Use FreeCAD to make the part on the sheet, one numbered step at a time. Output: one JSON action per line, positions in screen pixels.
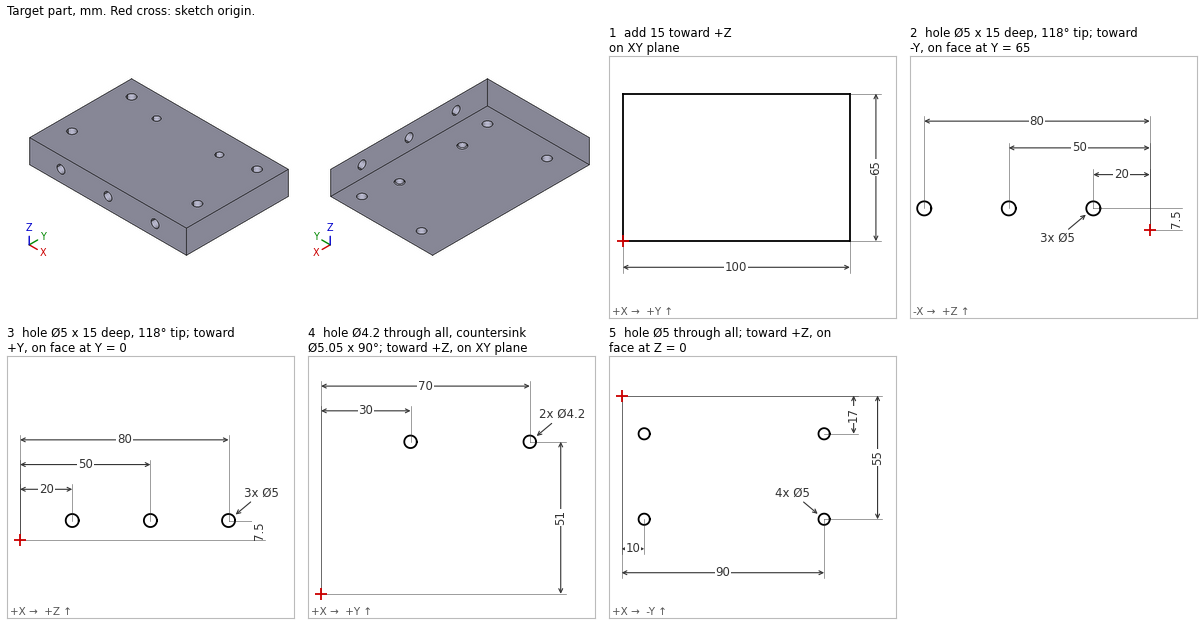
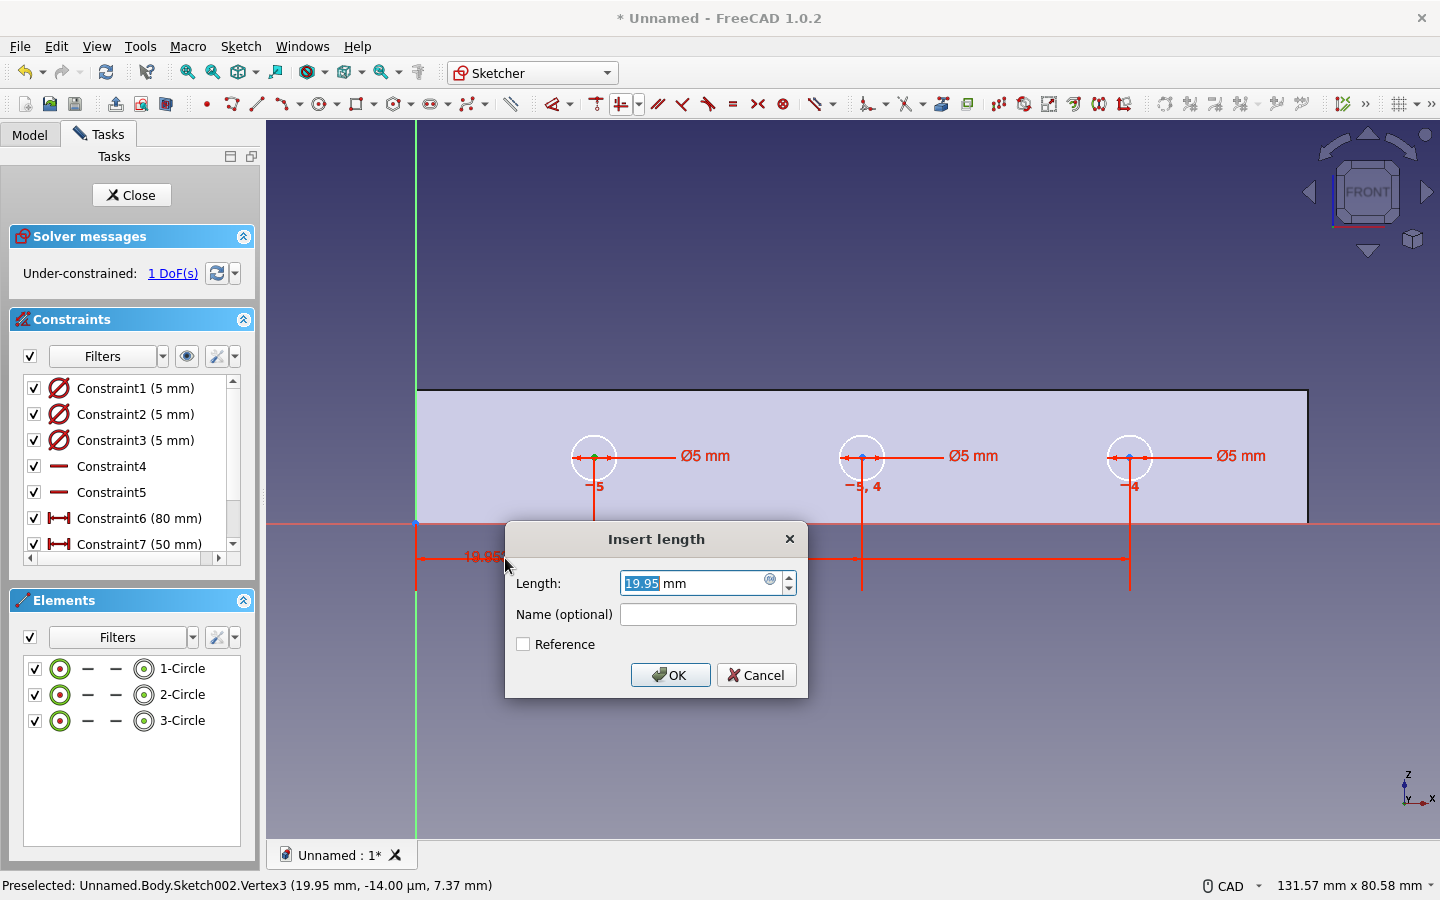
{"action": "type", "text": "20"}
{"action": "key", "text": "Return"}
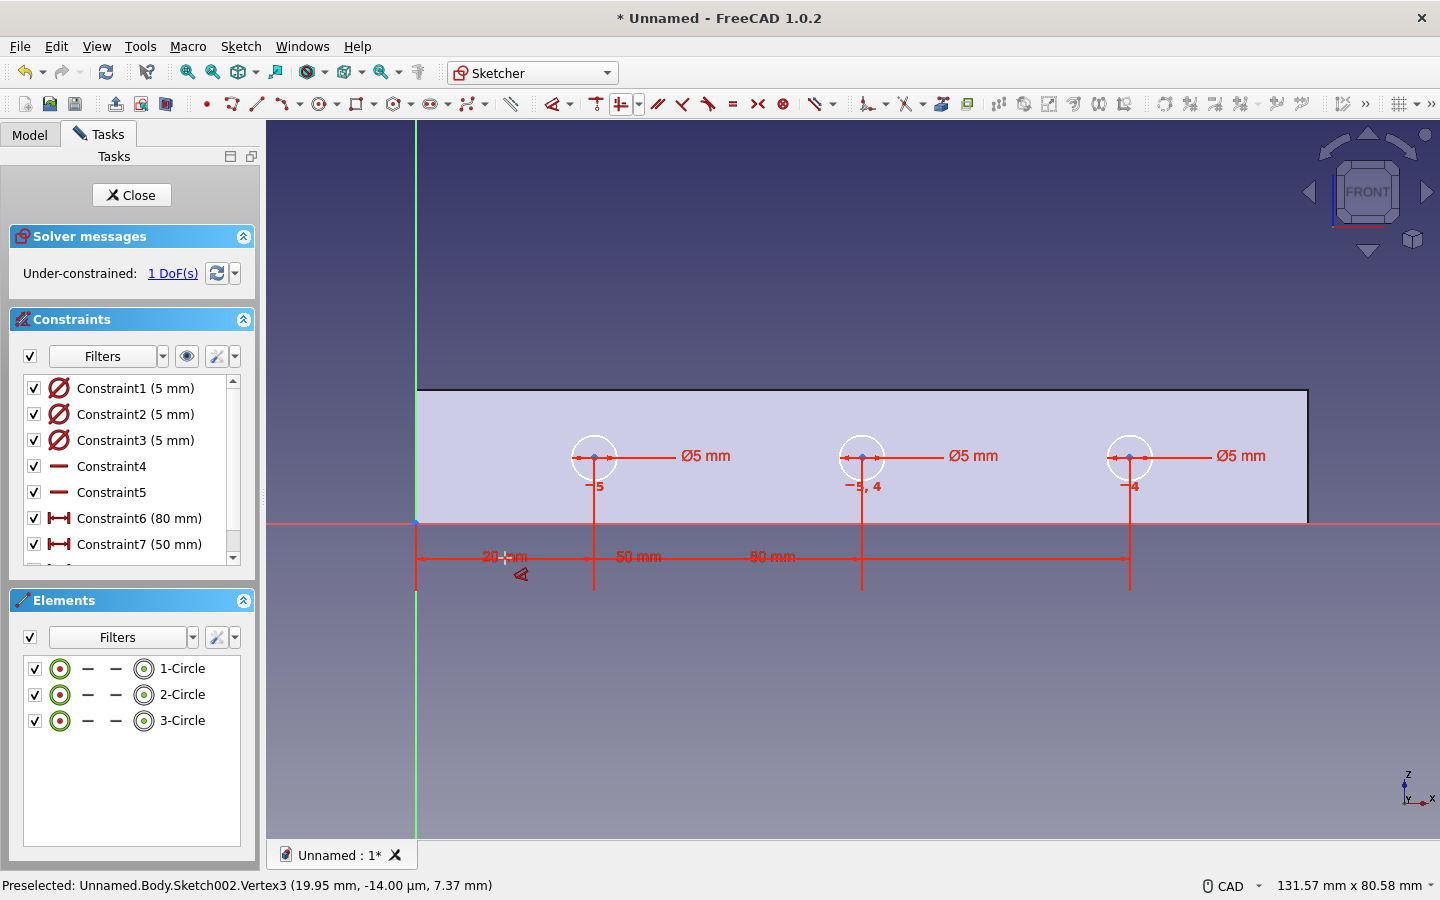
{"action": "left_click", "coordinate": [1130, 458]}
{"action": "left_click", "coordinate": [382, 491]}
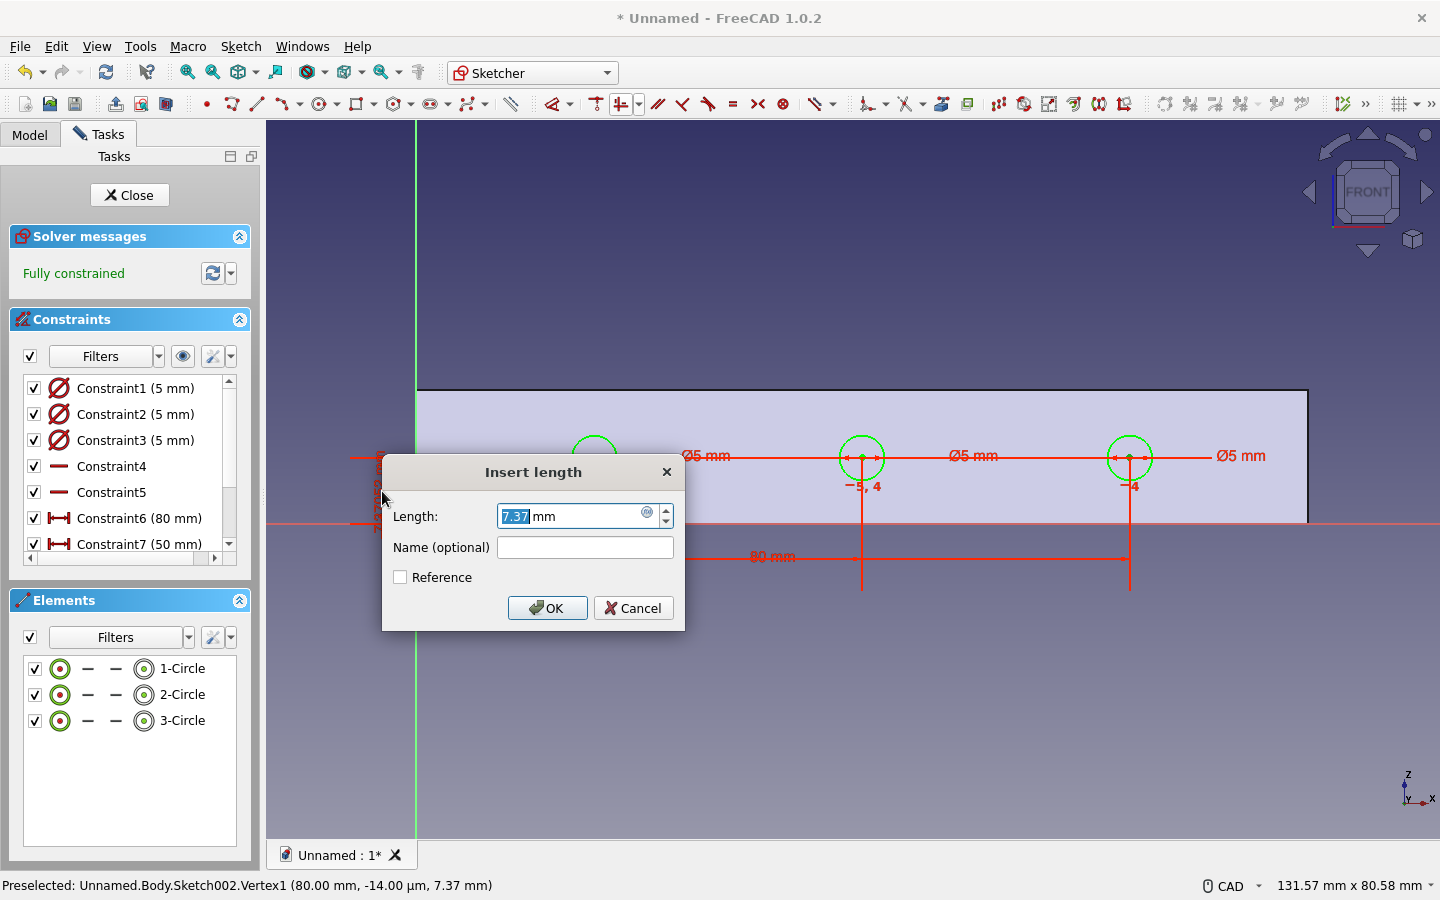
{"action": "type", "text": "7.5"}
{"action": "key", "text": "Return"}
{"action": "key", "text": "Escape"}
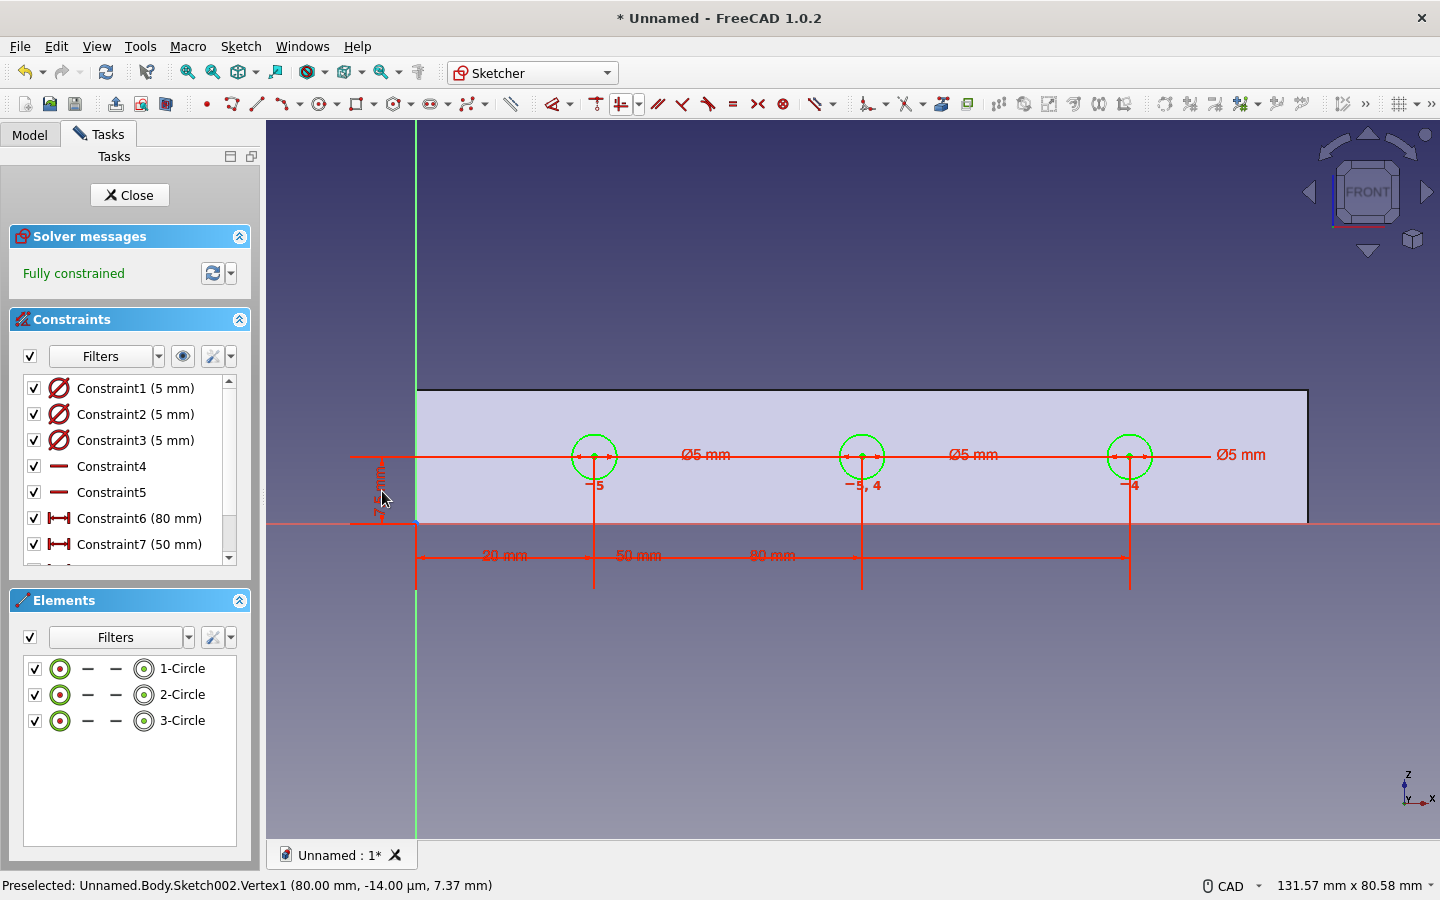
{"action": "left_click", "coordinate": [130, 195]}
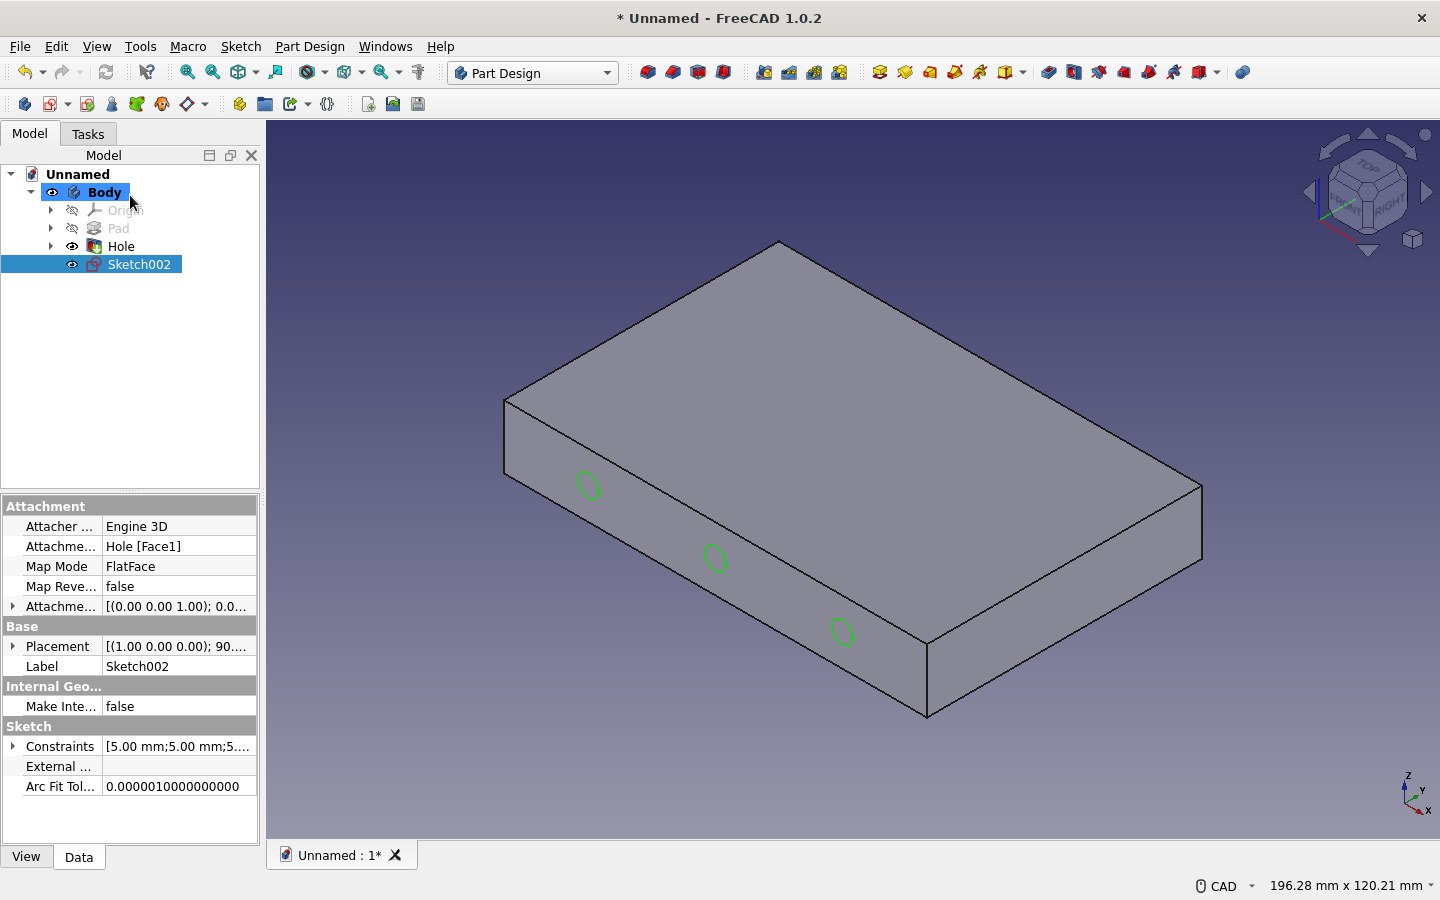
{"action": "left_click", "coordinate": [1074, 72]}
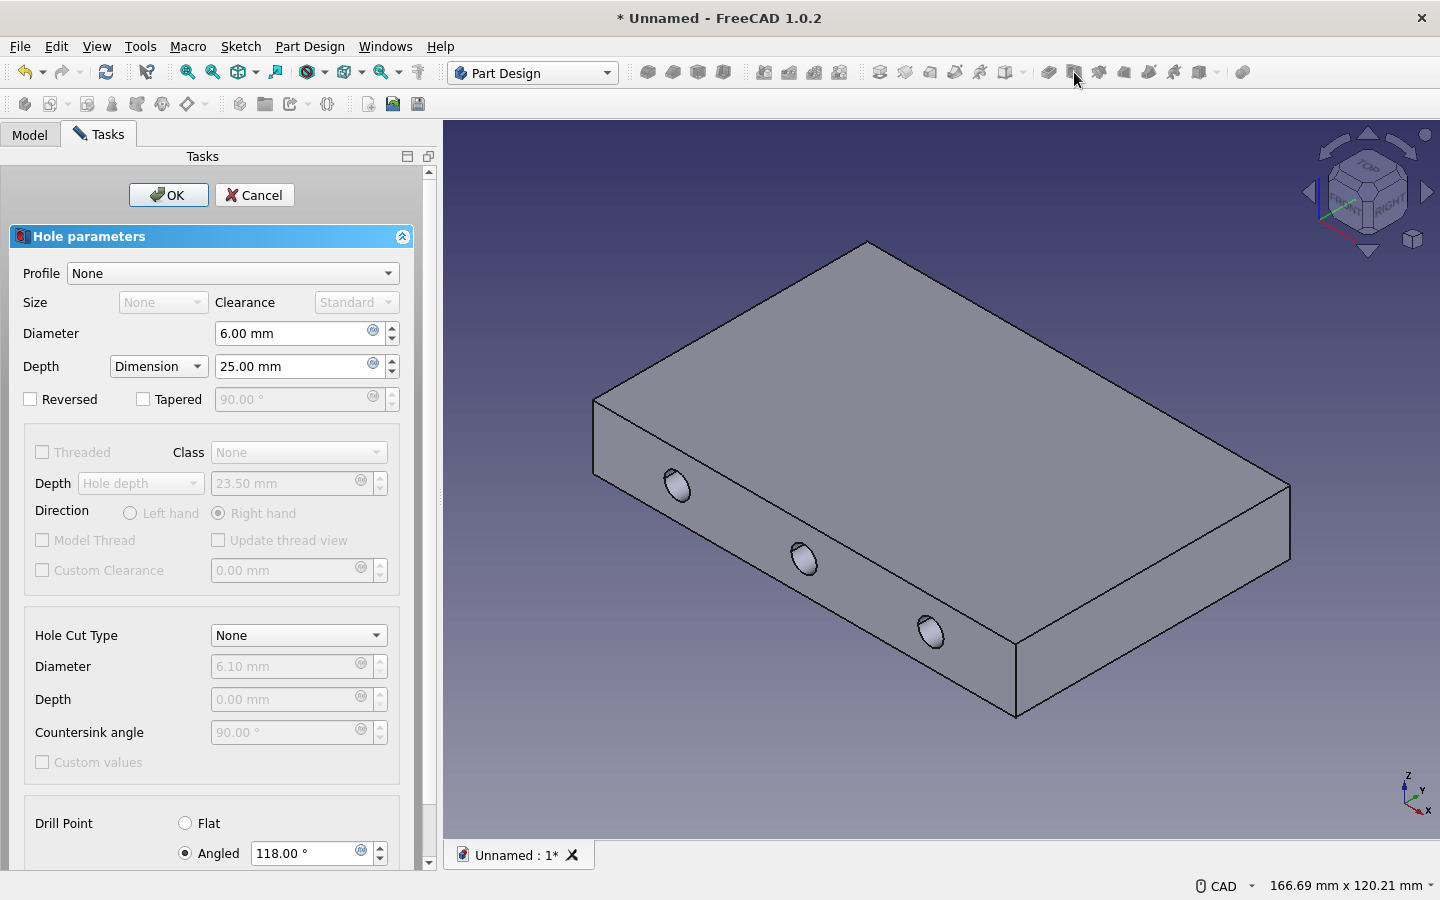
{"action": "triple_click", "coordinate": [300, 334]}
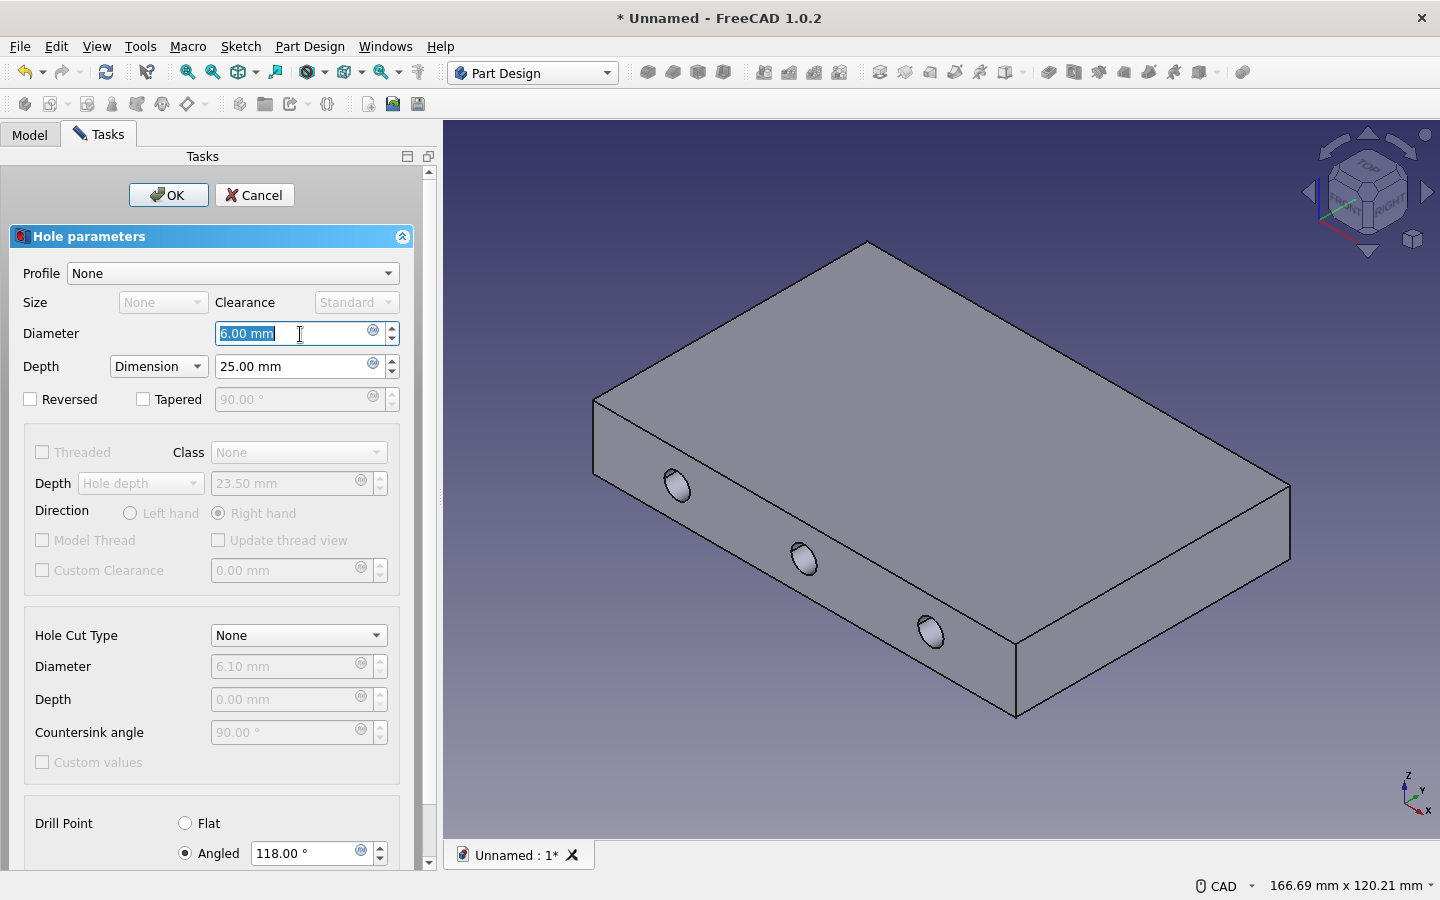
{"action": "type", "text": "5"}
{"action": "key", "text": "Tab"}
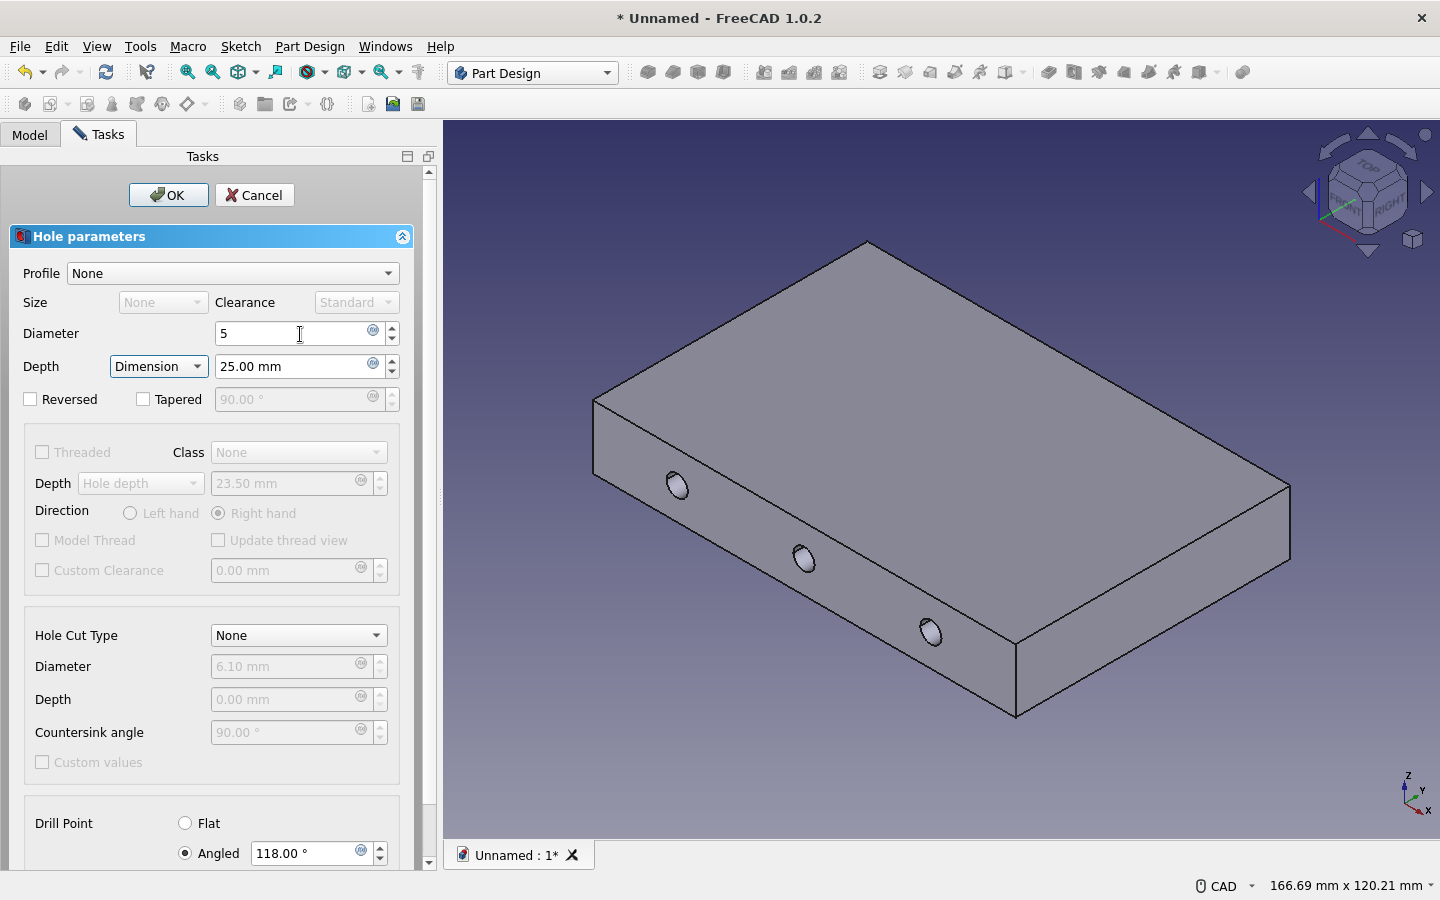
{"action": "triple_click", "coordinate": [300, 366]}